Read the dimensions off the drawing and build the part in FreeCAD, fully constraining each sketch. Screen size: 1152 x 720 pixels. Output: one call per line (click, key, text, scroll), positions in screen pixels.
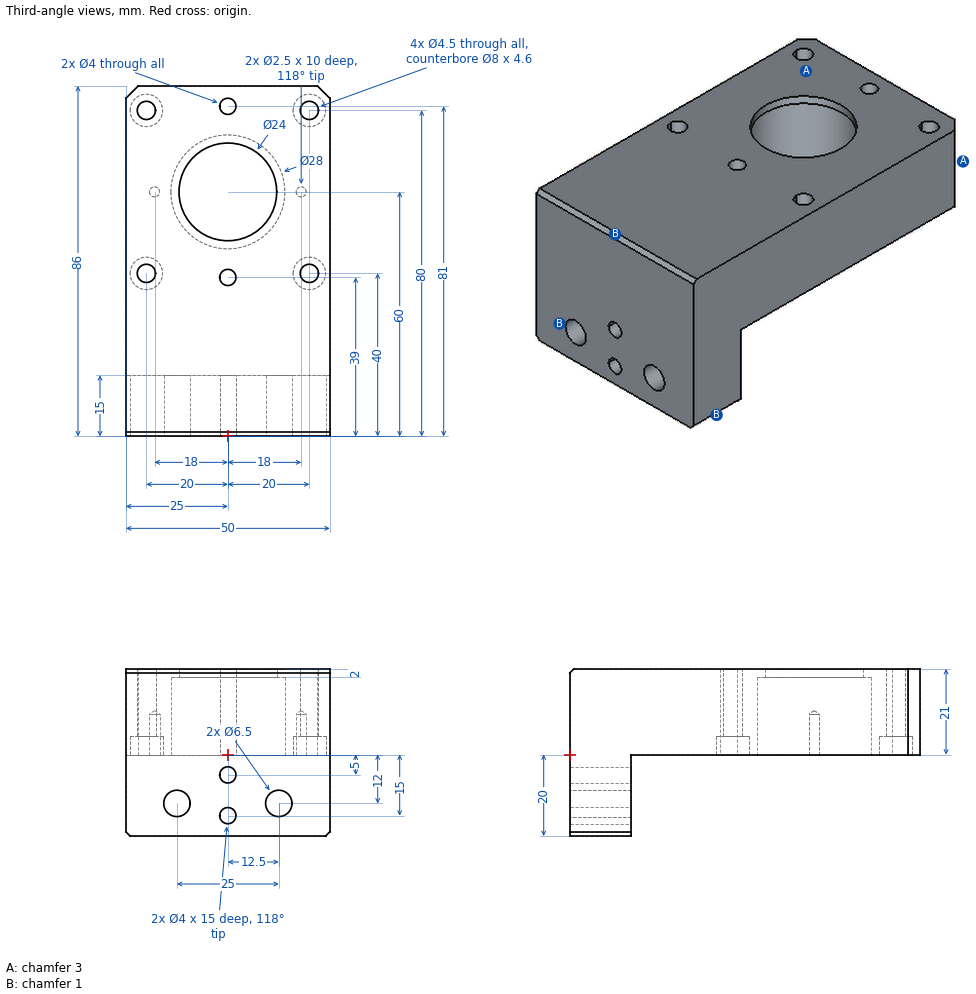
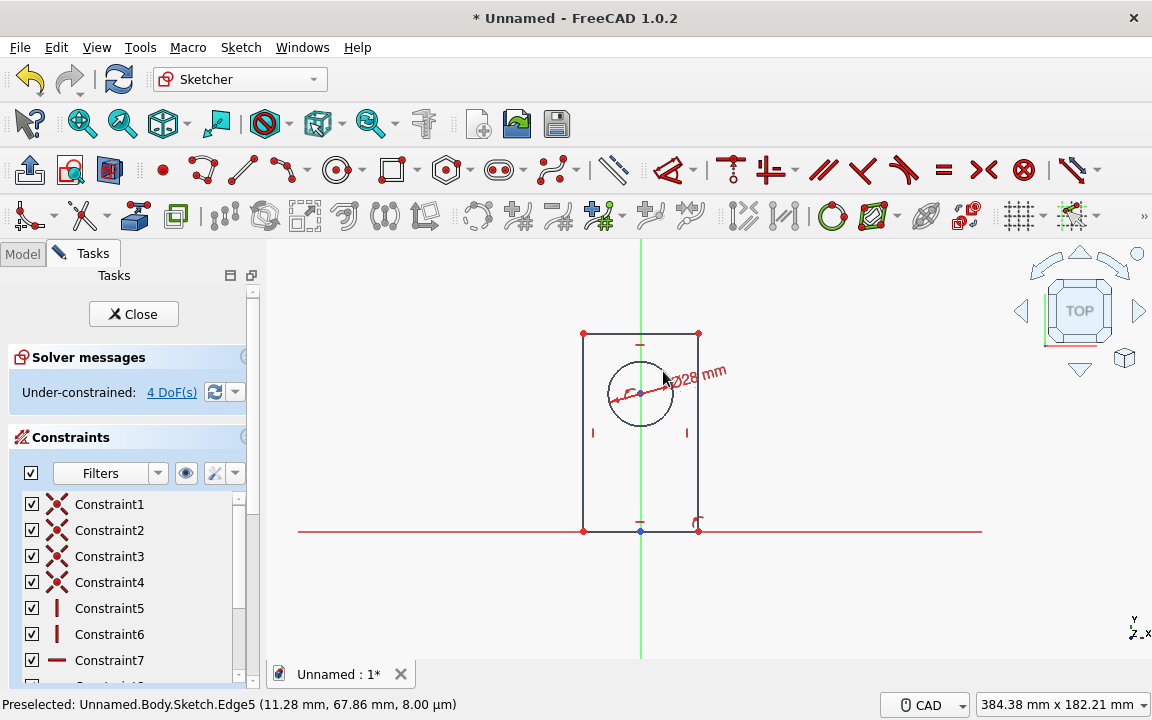
click(583, 393)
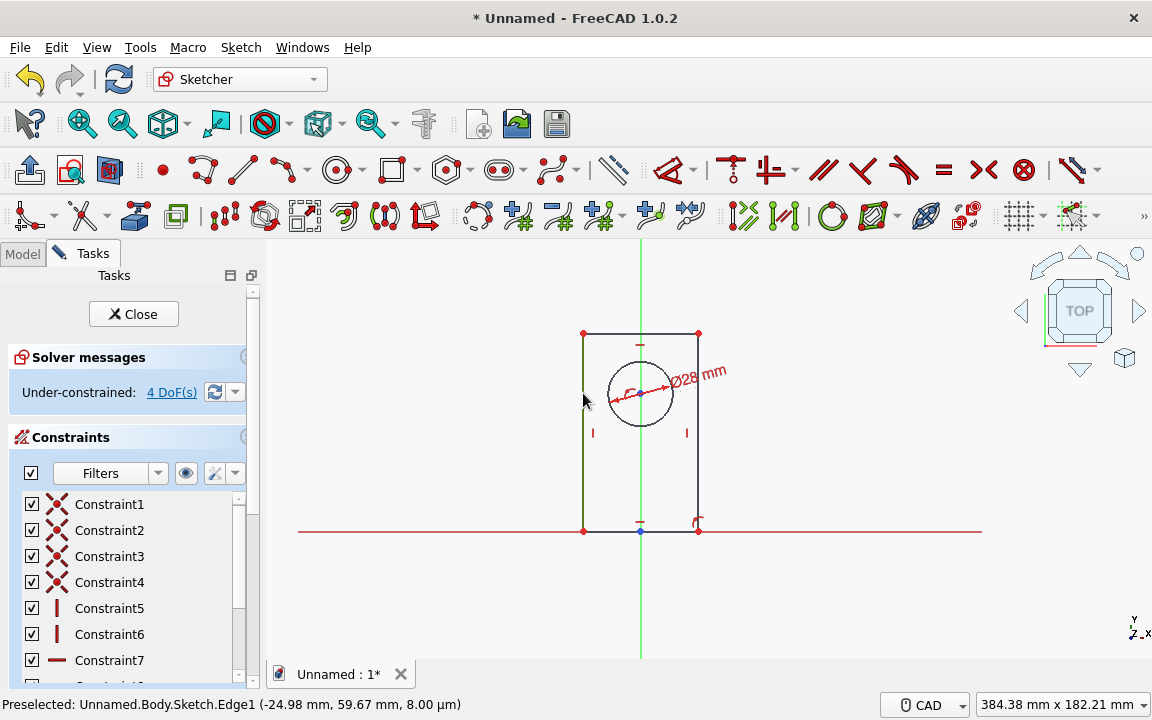
key(i)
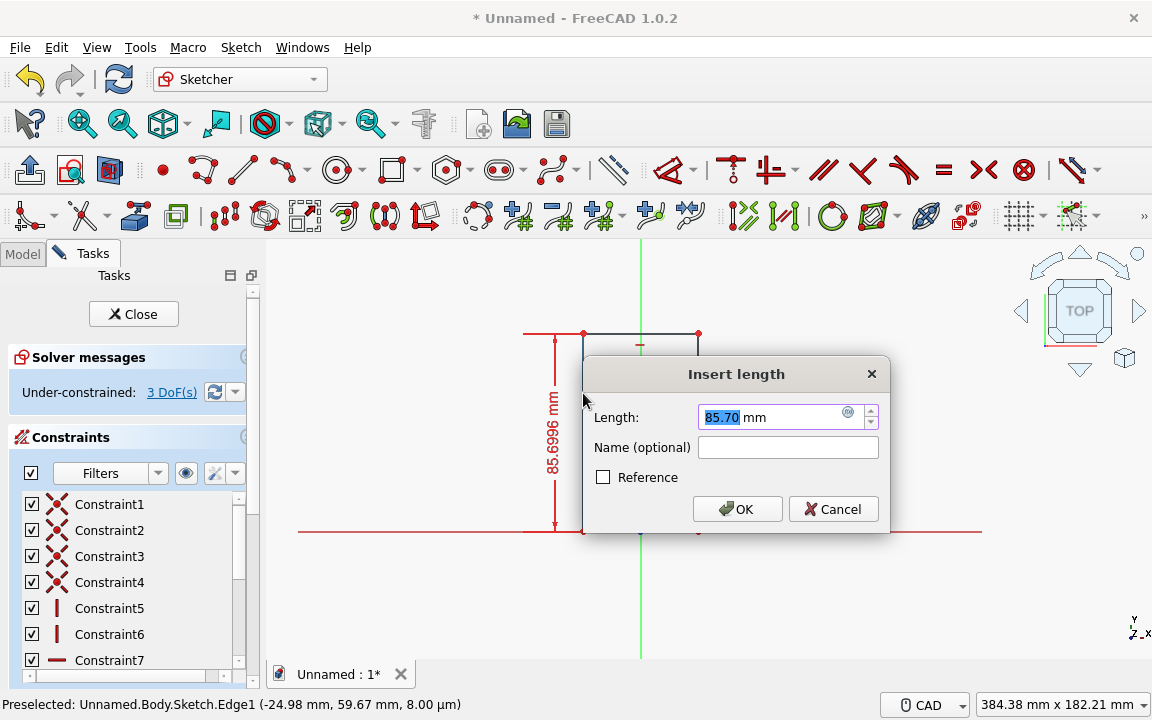
text(86)
key(Return)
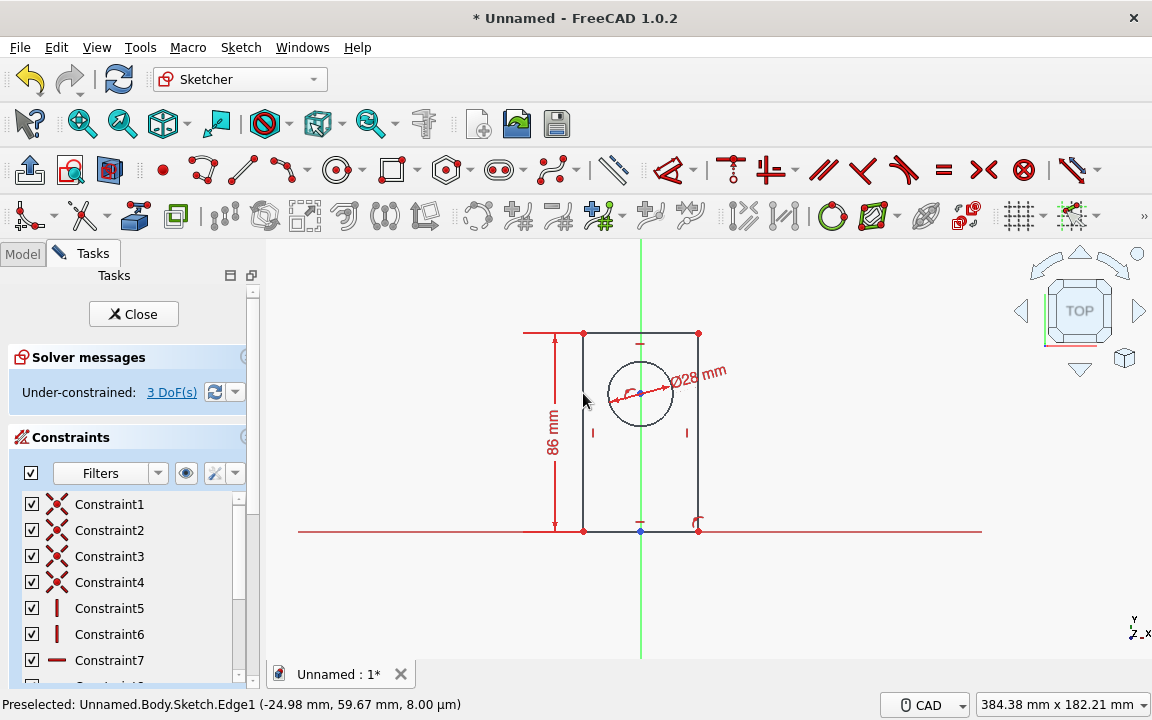
click(618, 532)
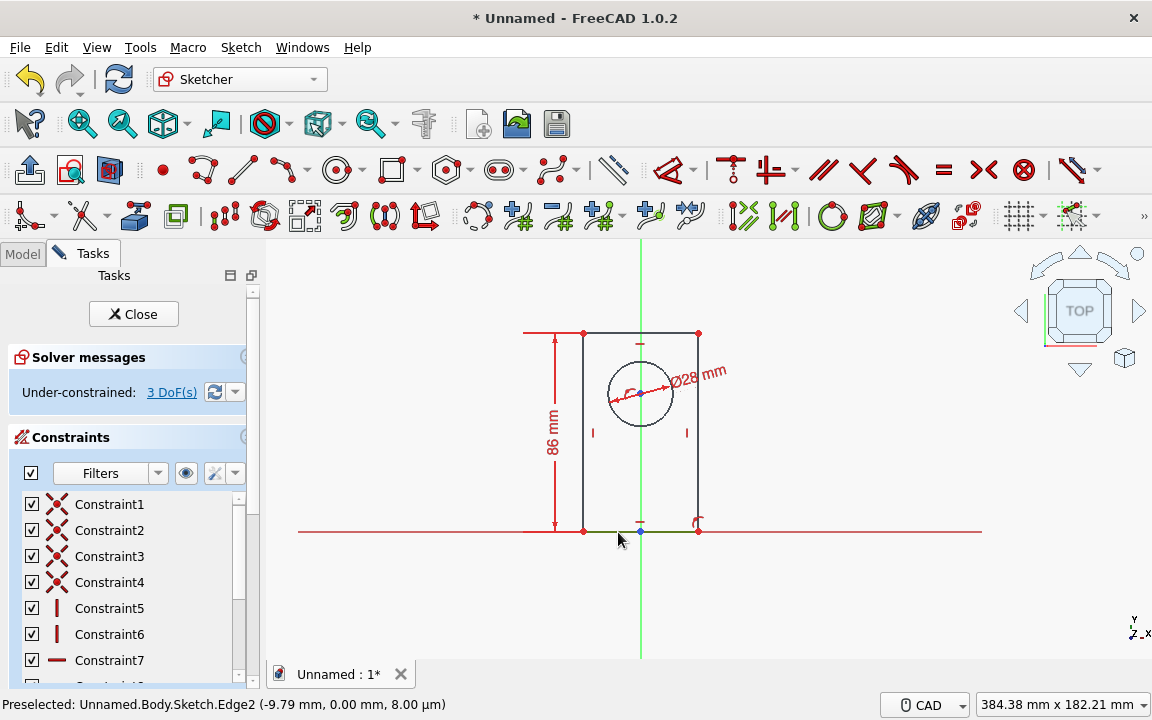
key(l)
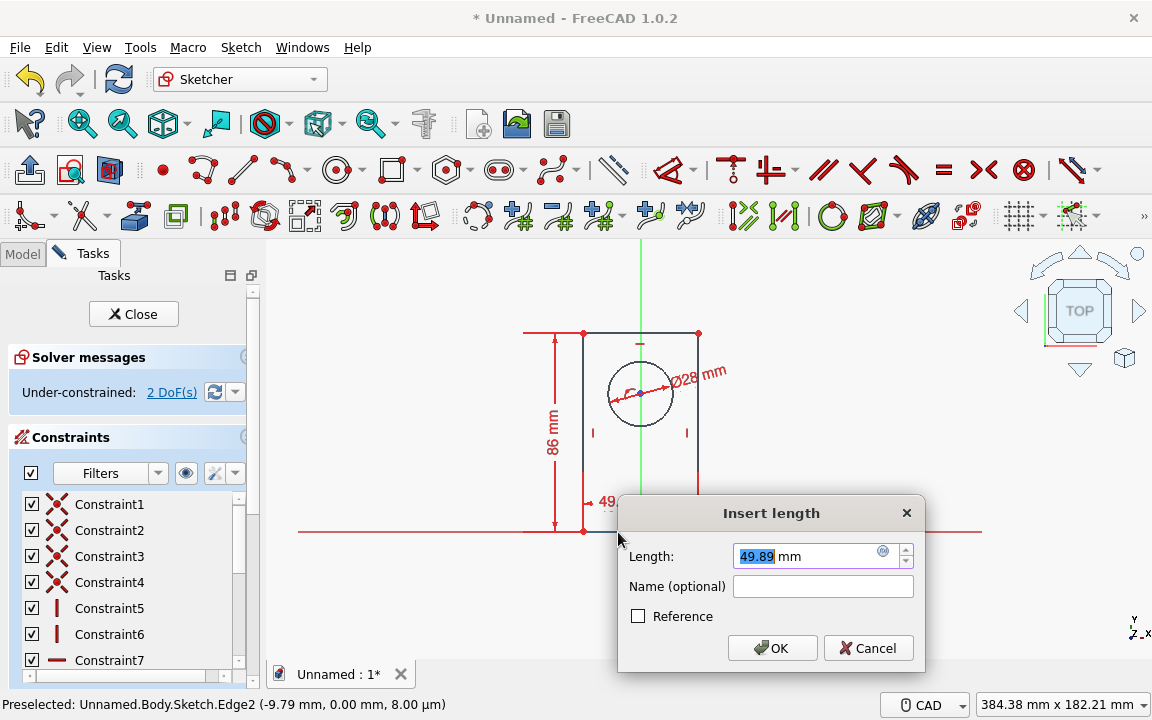
text(50)
key(Return)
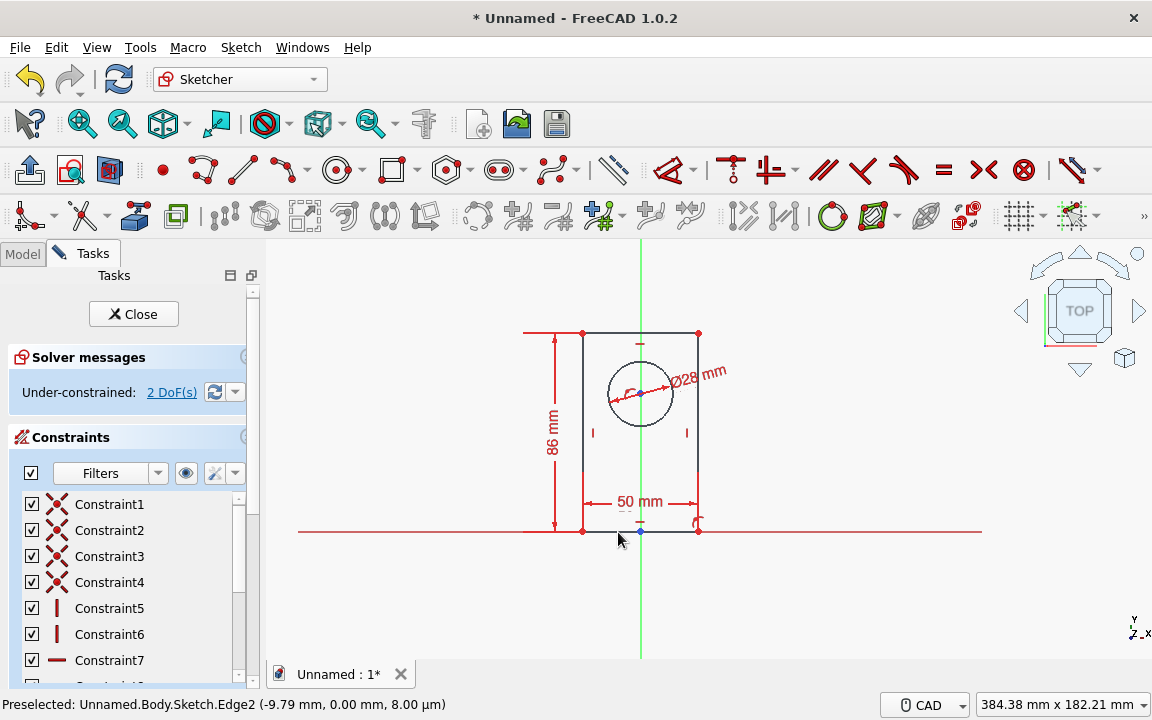
click(641, 394)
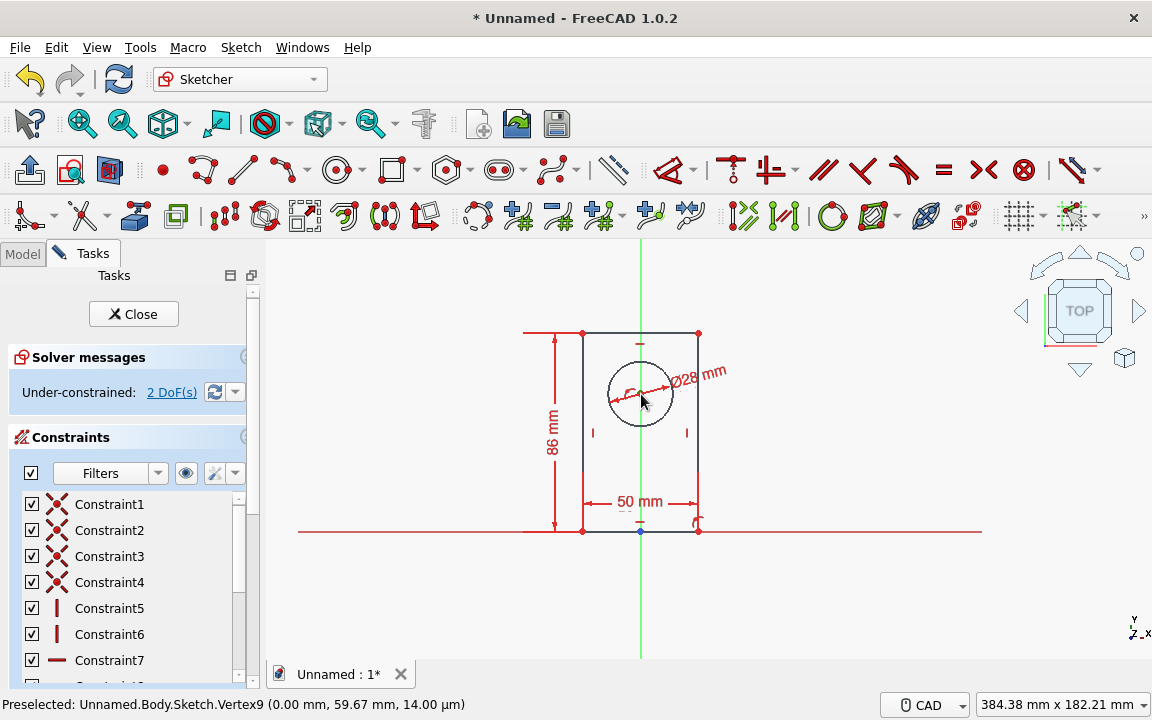
key(i)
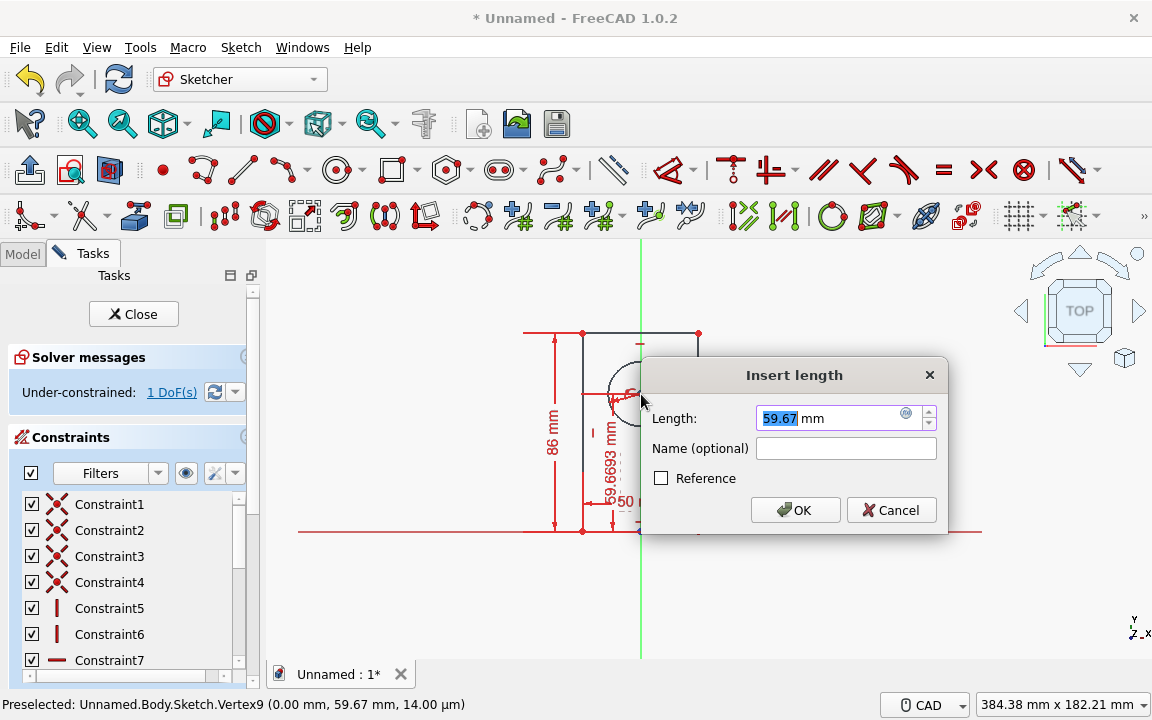
text(60)
key(Return)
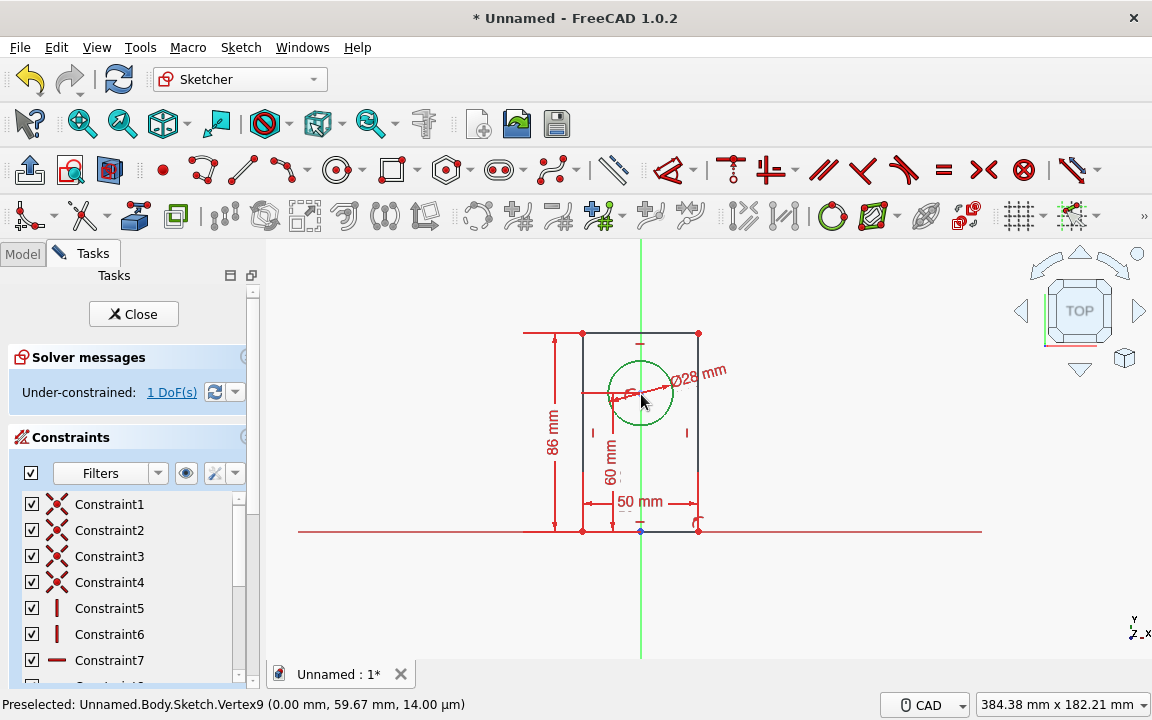
click(583, 333)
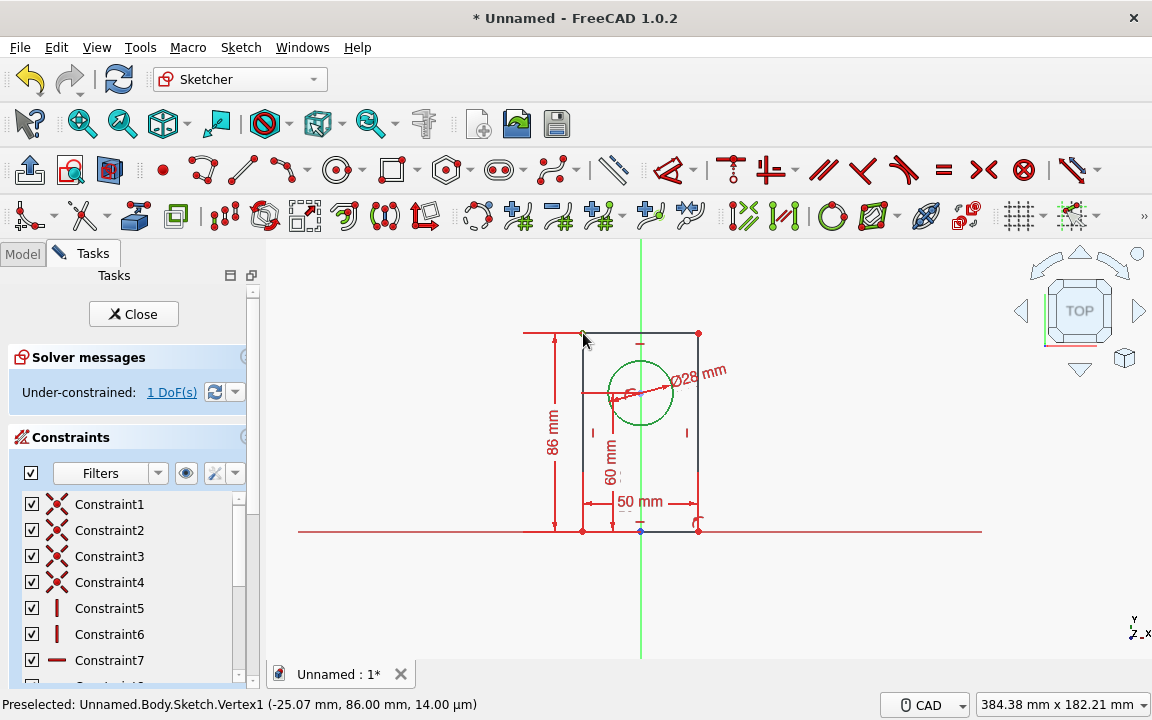
key(l)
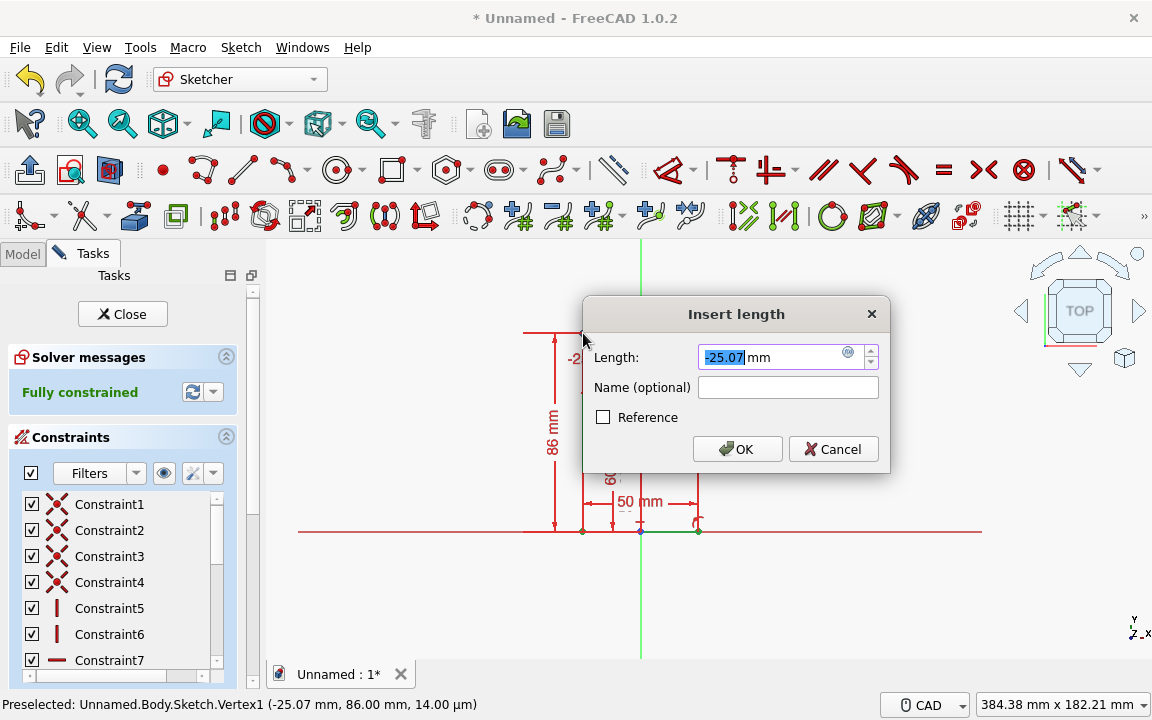
text(-25)
key(Return)